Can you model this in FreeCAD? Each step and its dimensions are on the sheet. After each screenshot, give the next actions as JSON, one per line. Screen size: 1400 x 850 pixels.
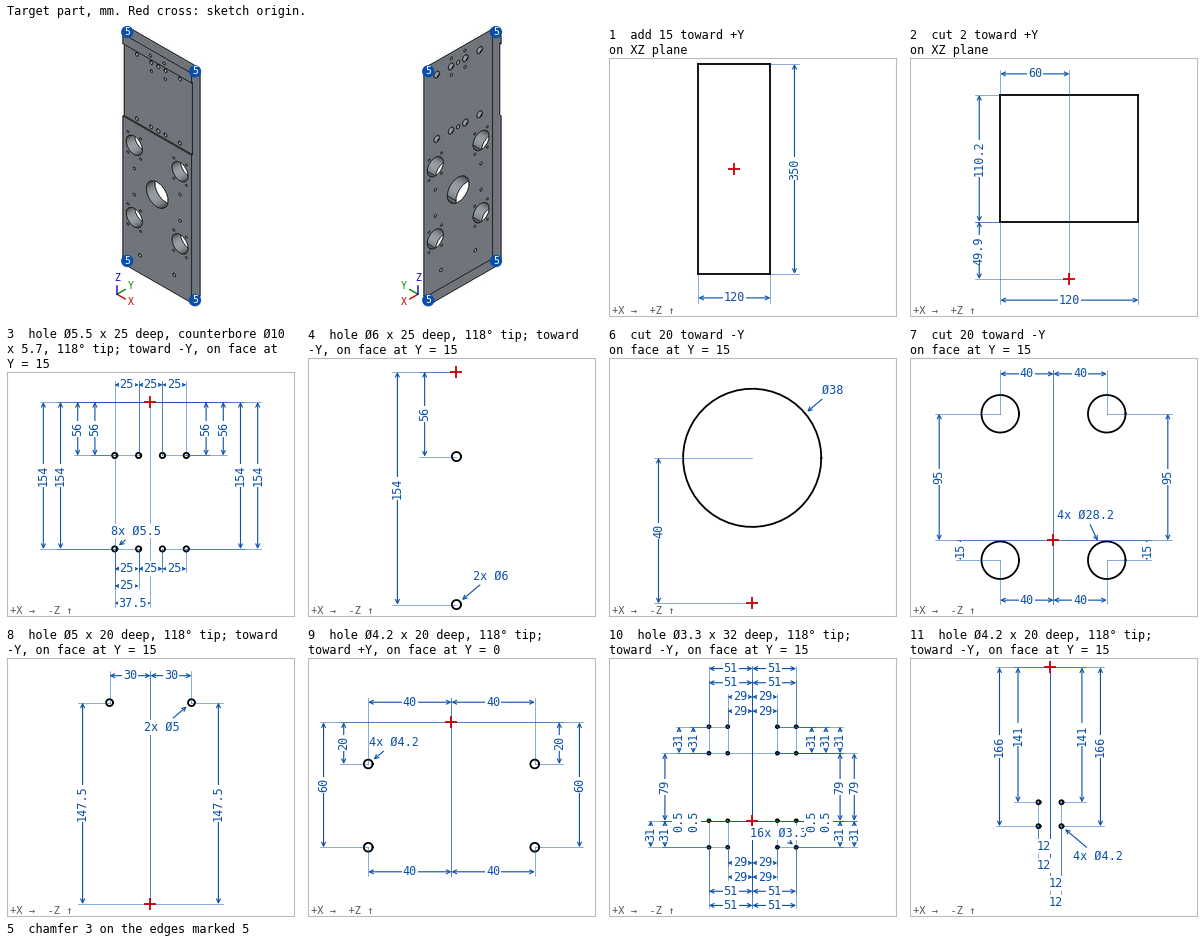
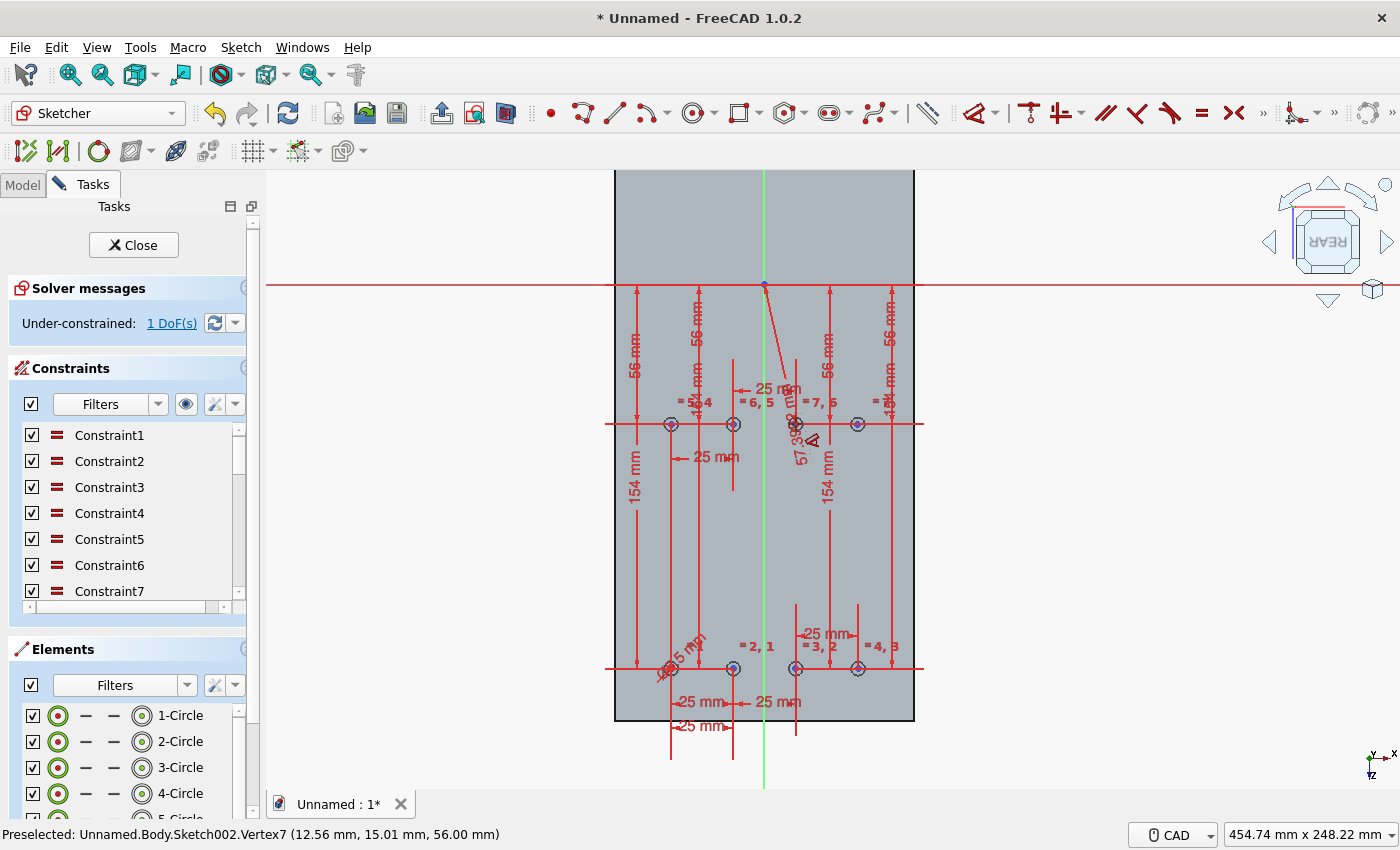
{"action": "left_click", "coordinate": [858, 424]}
{"action": "left_click", "coordinate": [827, 506]}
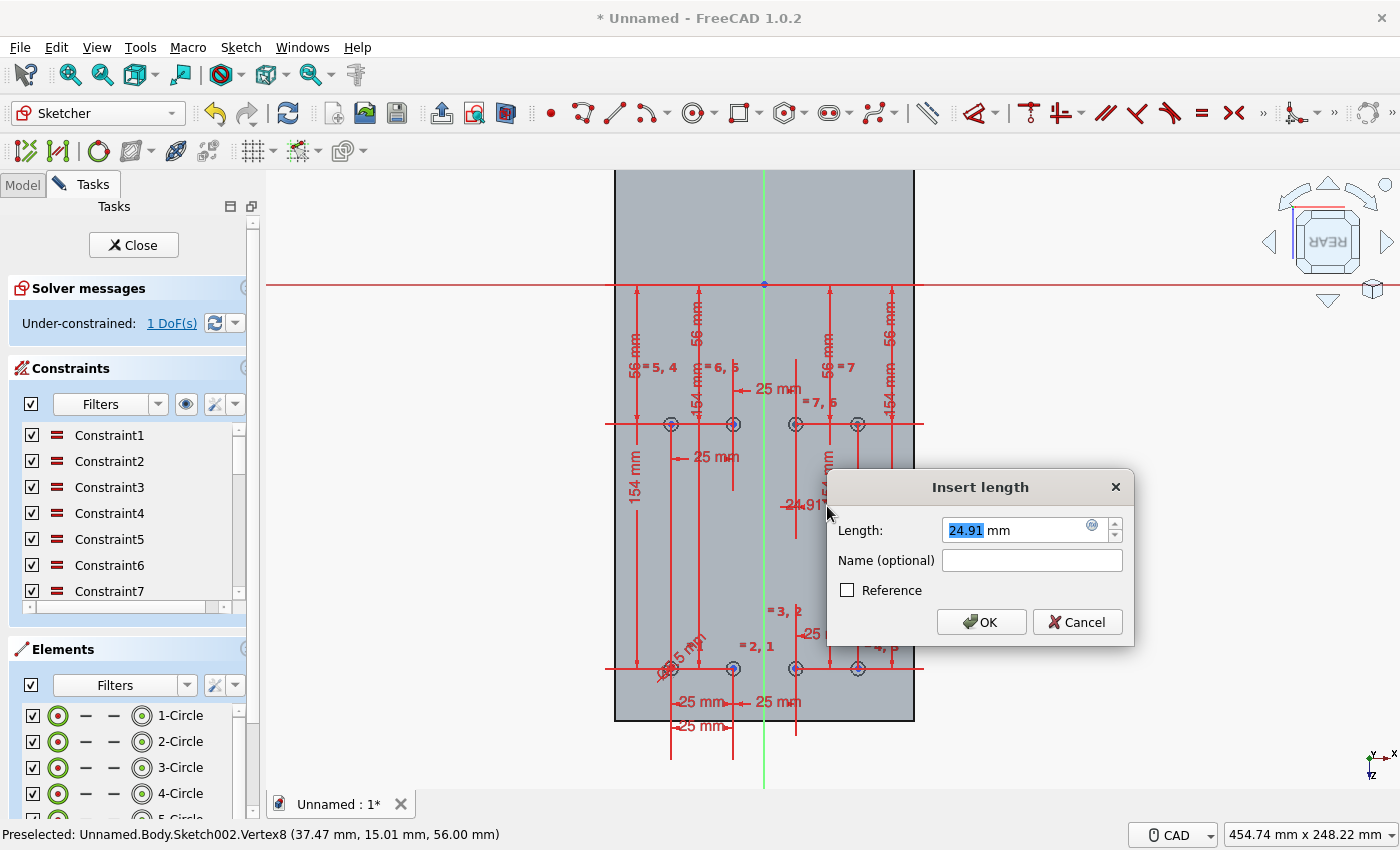
{"action": "type", "text": "25"}
{"action": "key", "text": "Return"}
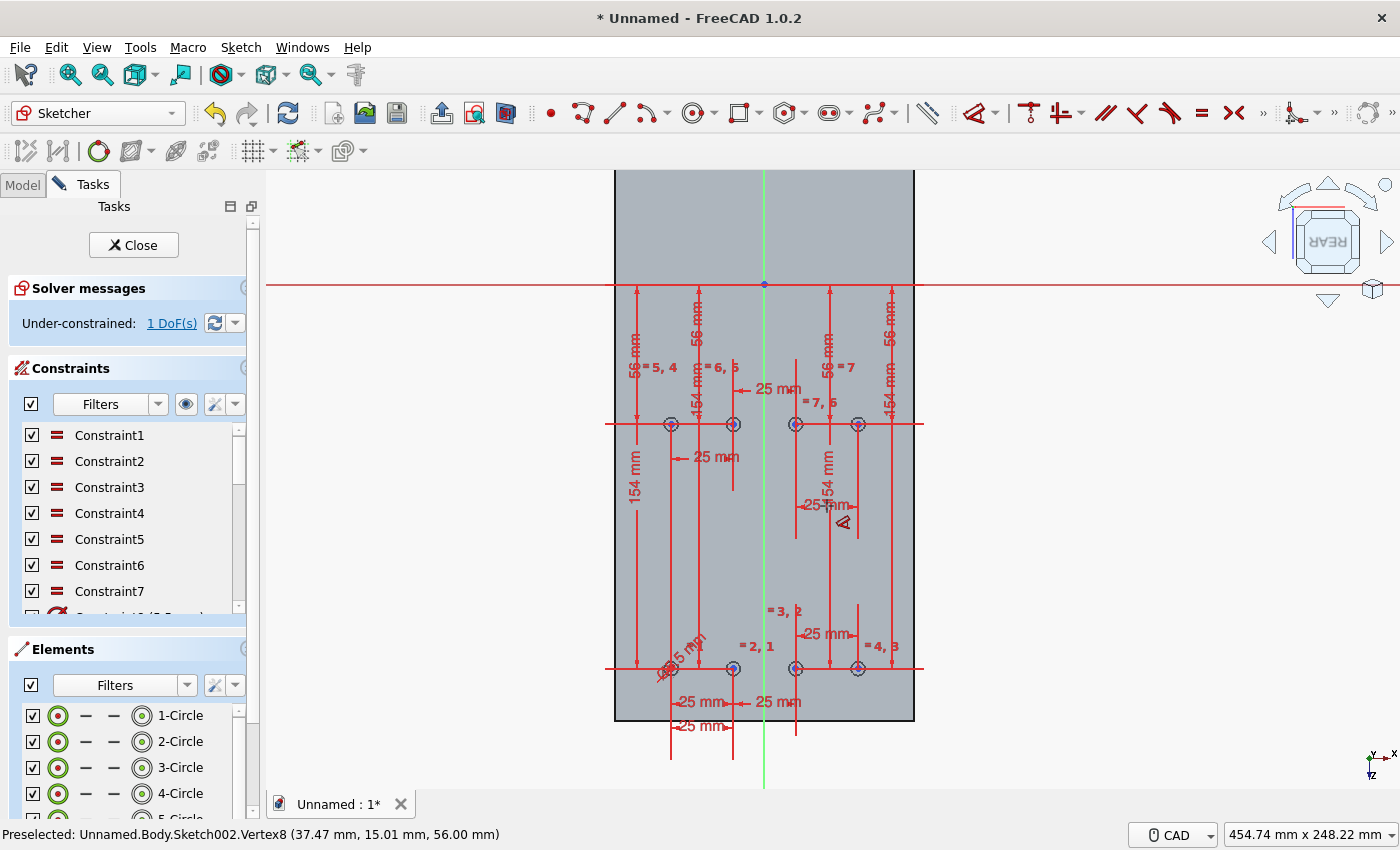
{"action": "left_click", "coordinate": [671, 669]}
{"action": "left_click", "coordinate": [718, 251]}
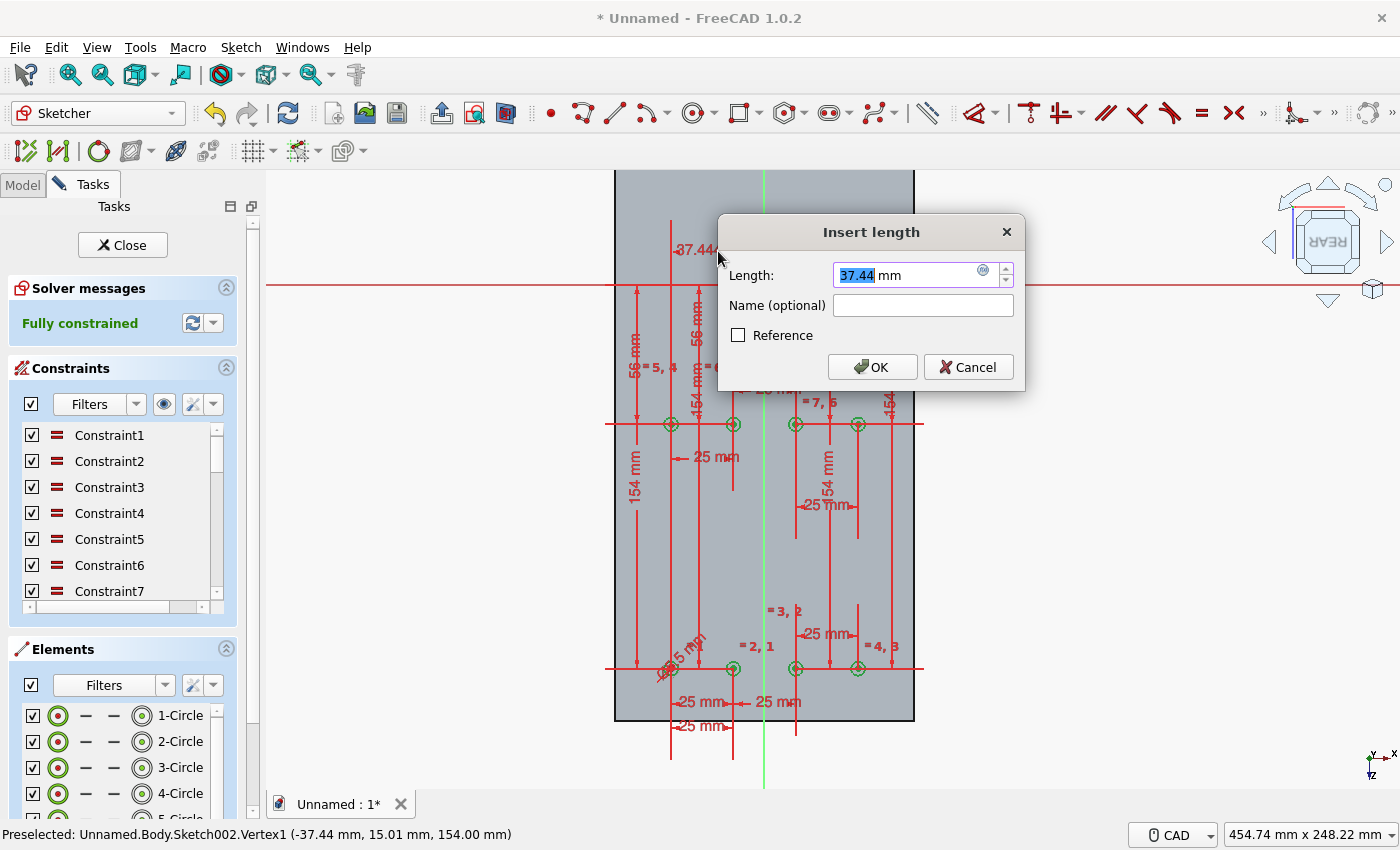
{"action": "type", "text": "37.5"}
{"action": "key", "text": "Return"}
{"action": "key", "text": "Escape"}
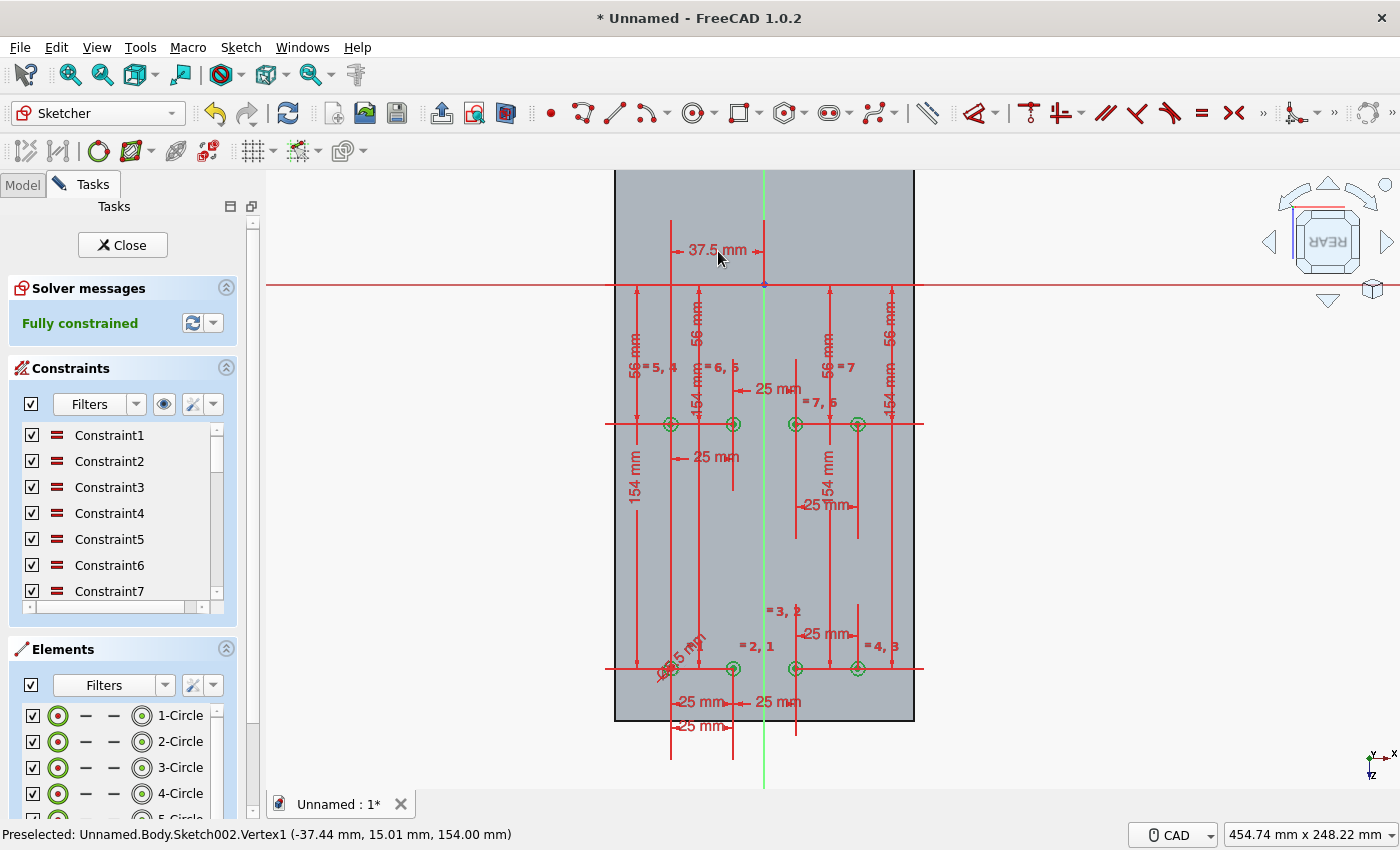
{"action": "left_click", "coordinate": [123, 245]}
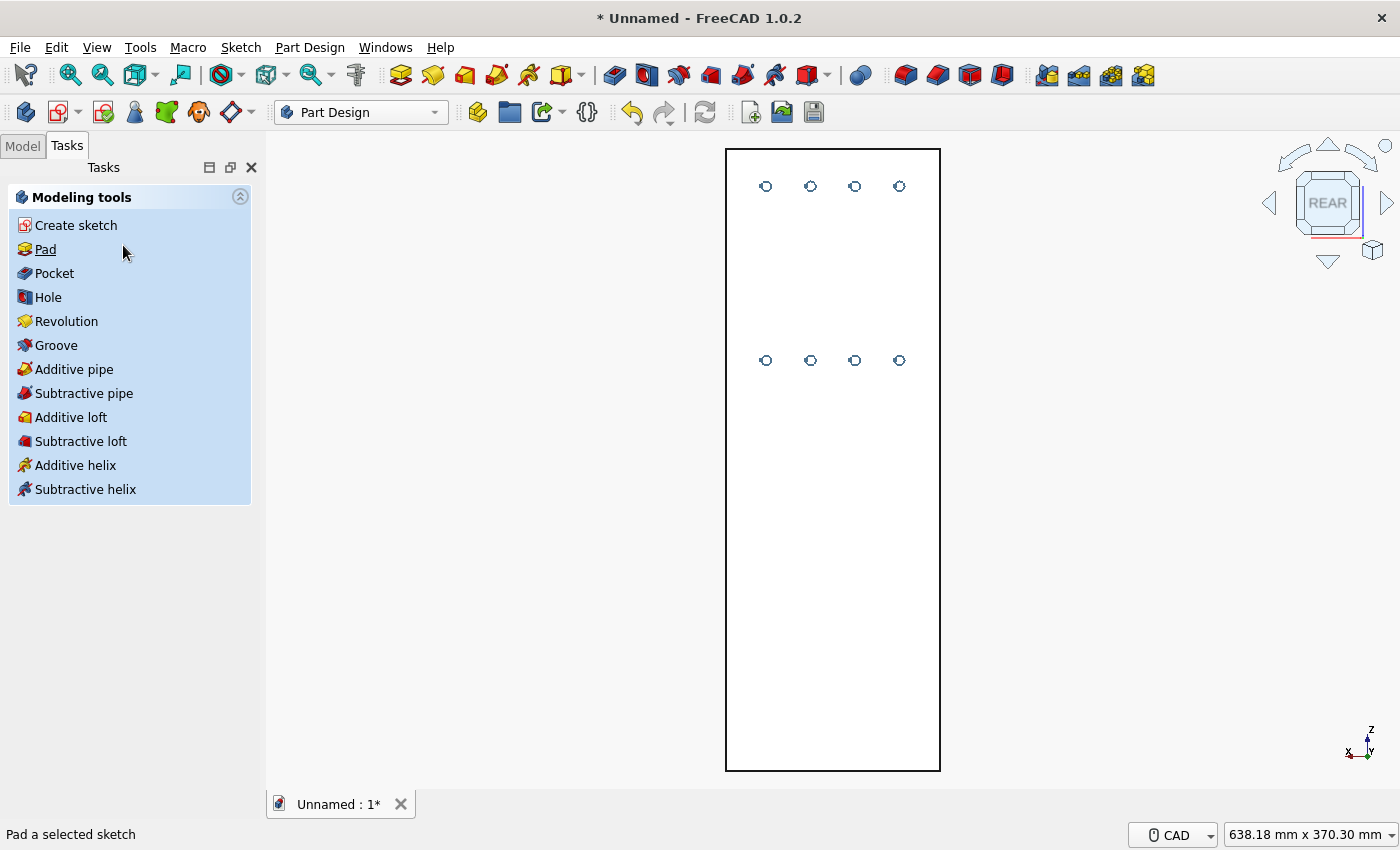
{"action": "left_click", "coordinate": [648, 76]}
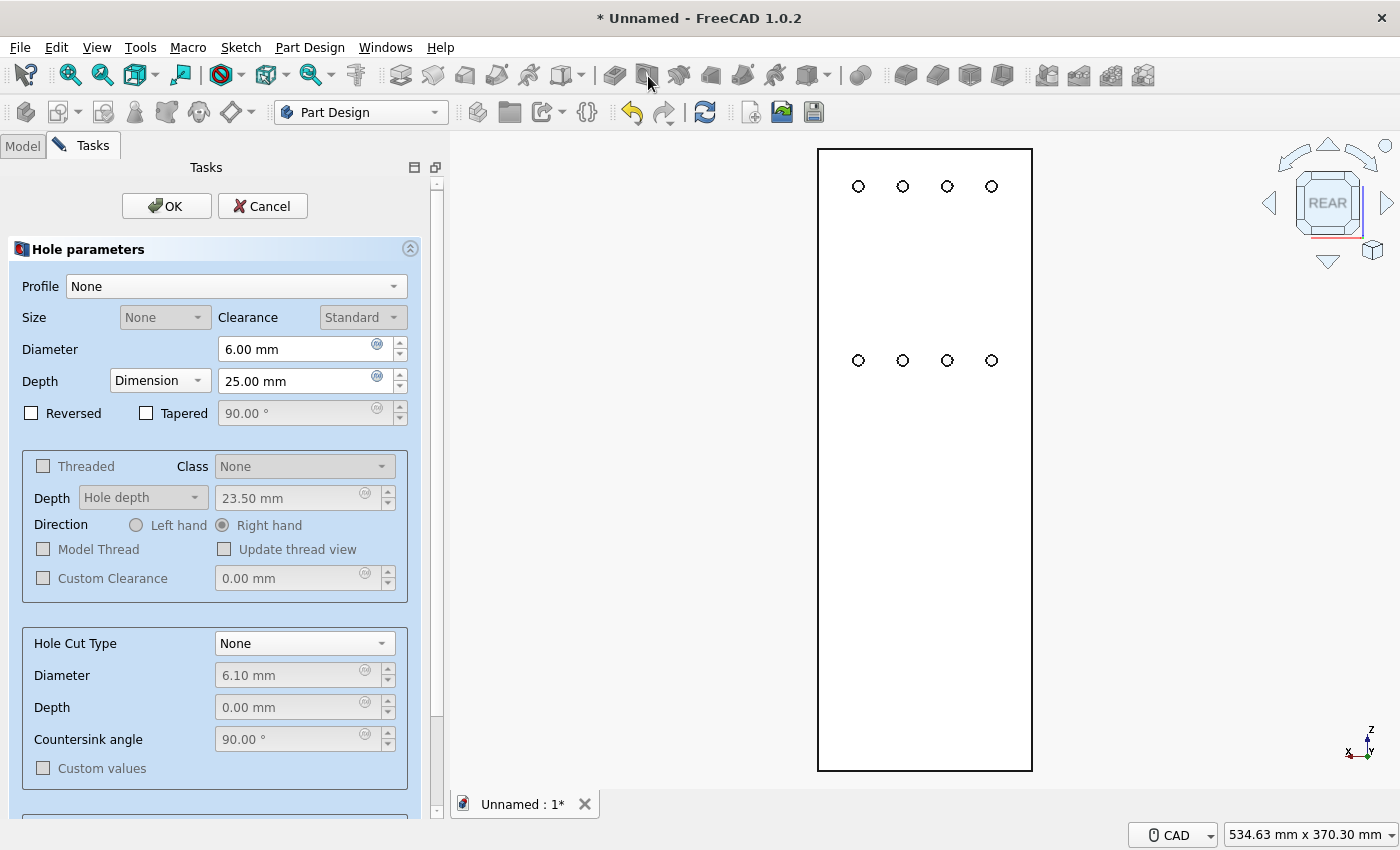
{"action": "triple_click", "coordinate": [305, 349]}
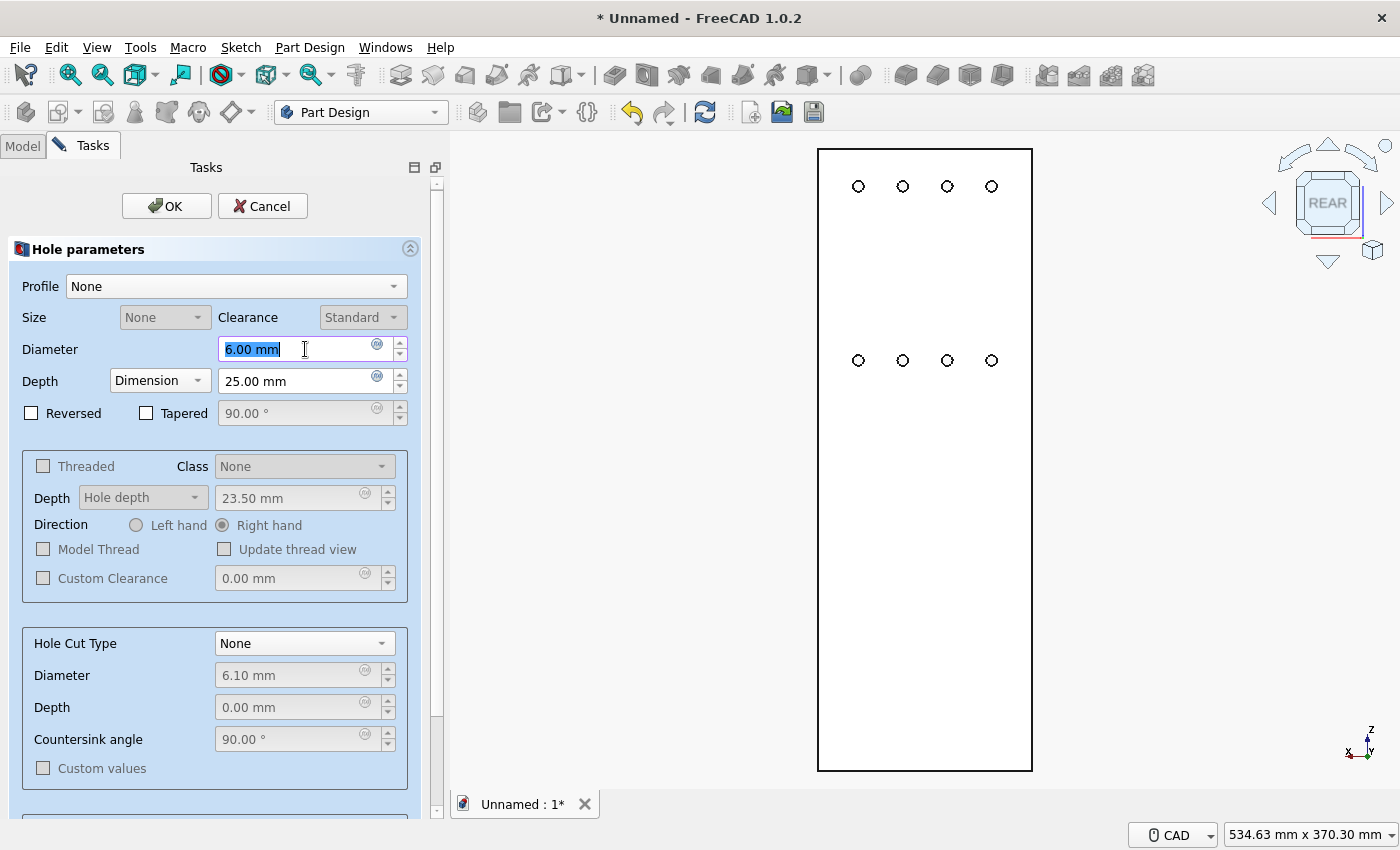
{"action": "type", "text": "5.5"}
{"action": "key", "text": "Tab"}